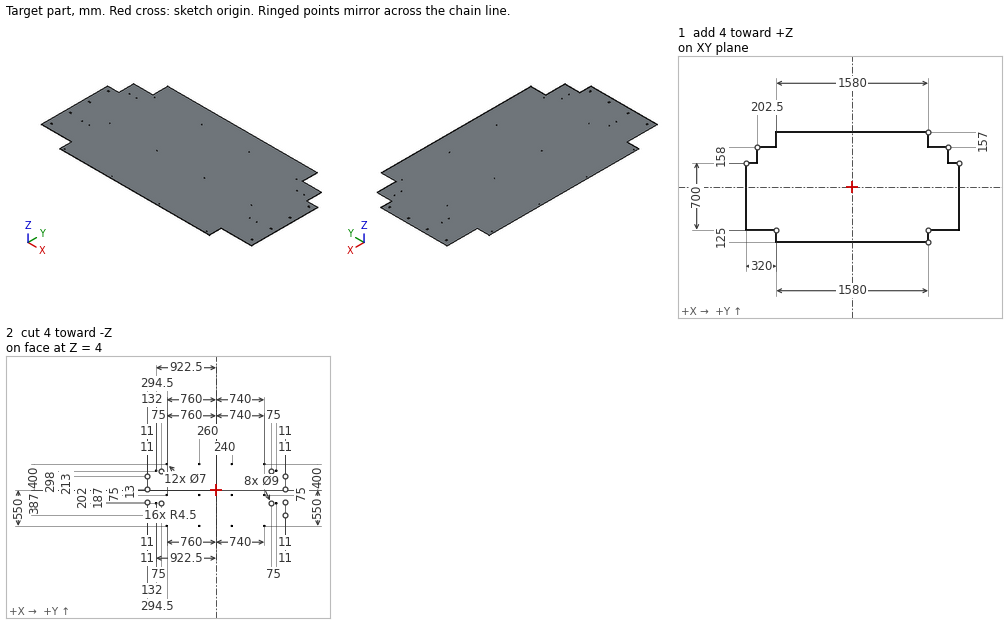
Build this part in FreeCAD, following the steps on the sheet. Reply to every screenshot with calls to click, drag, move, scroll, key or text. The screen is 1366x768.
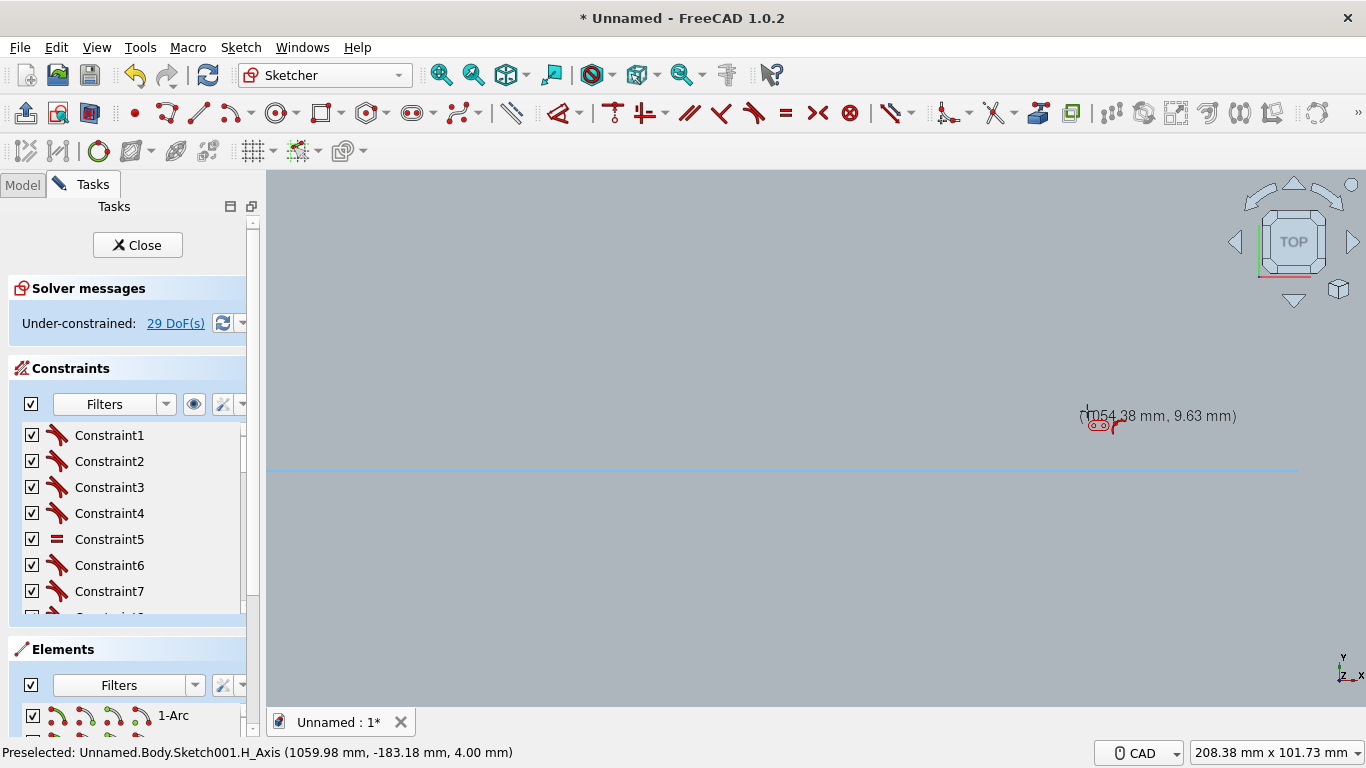
scroll(1087, 411, down, 14)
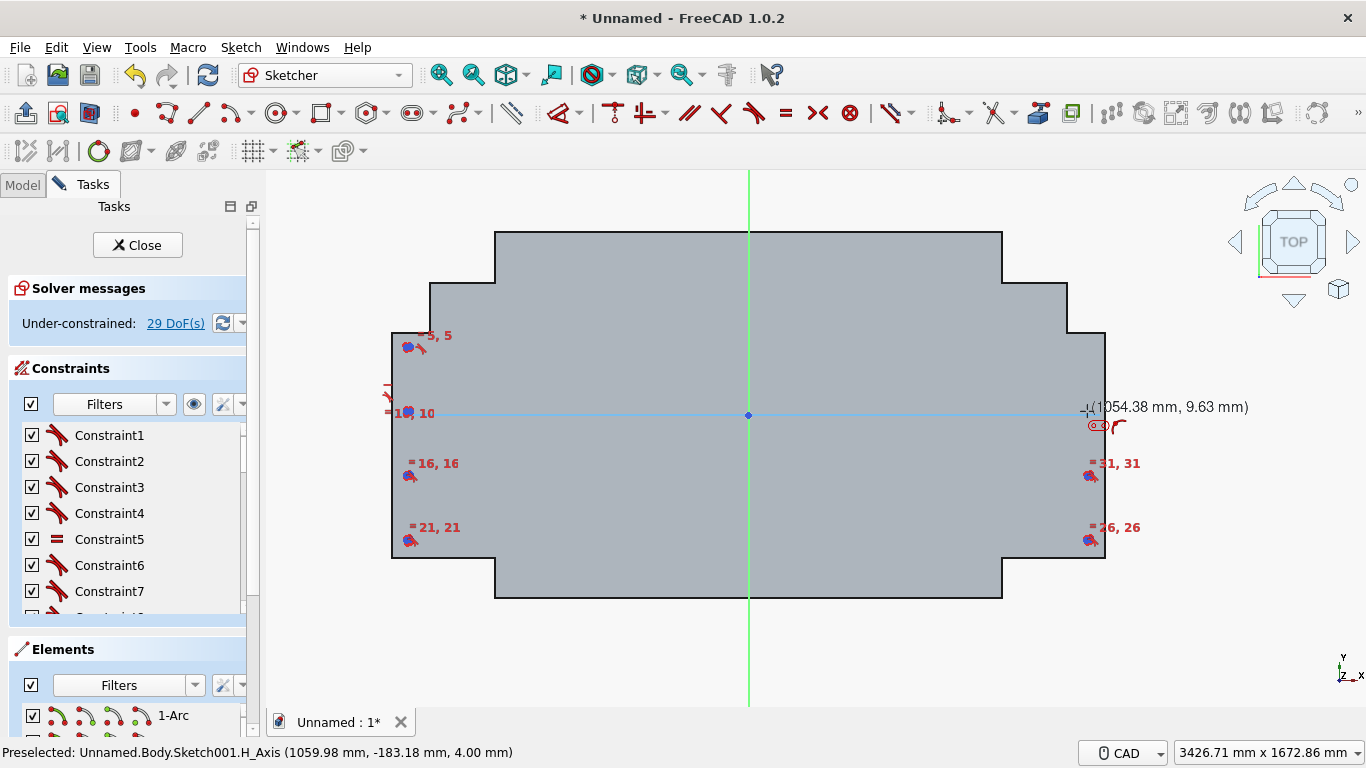
scroll(1087, 411, up, 7)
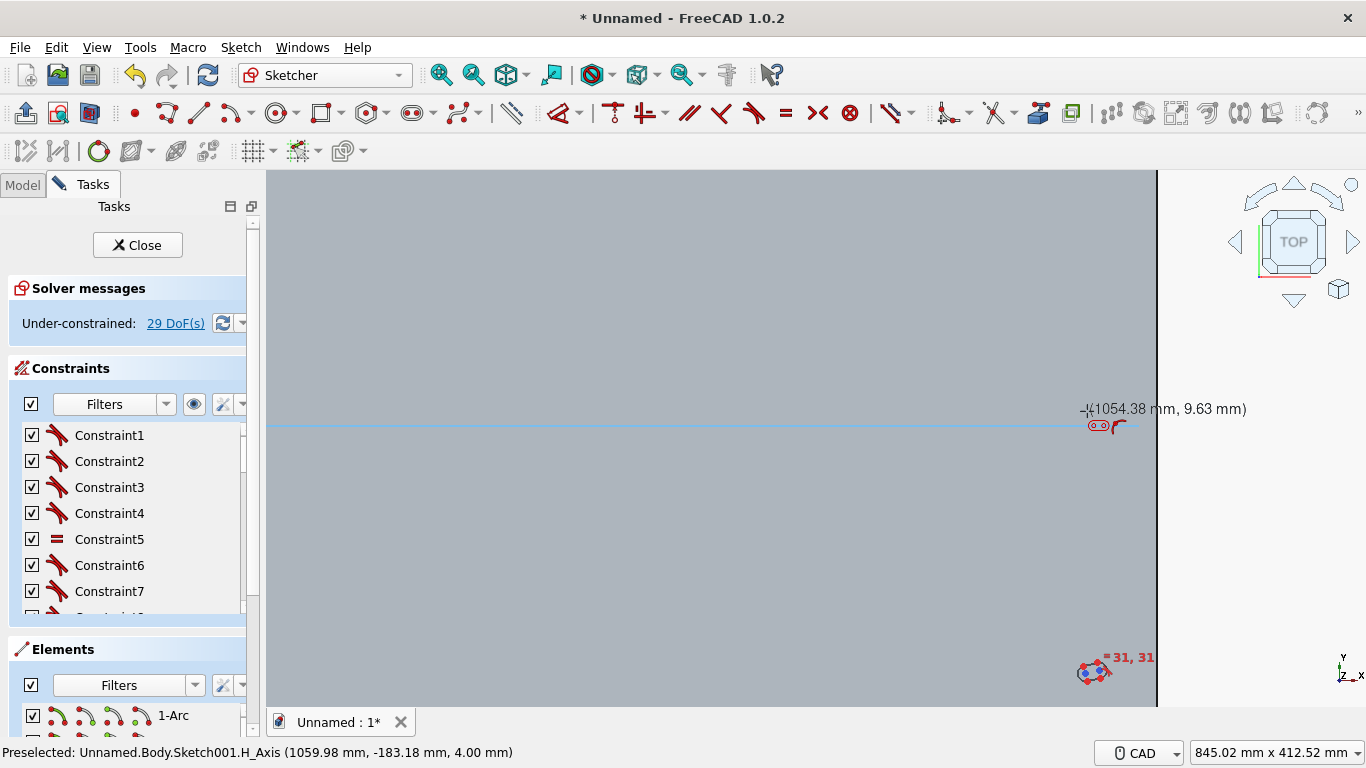
click(1085, 409)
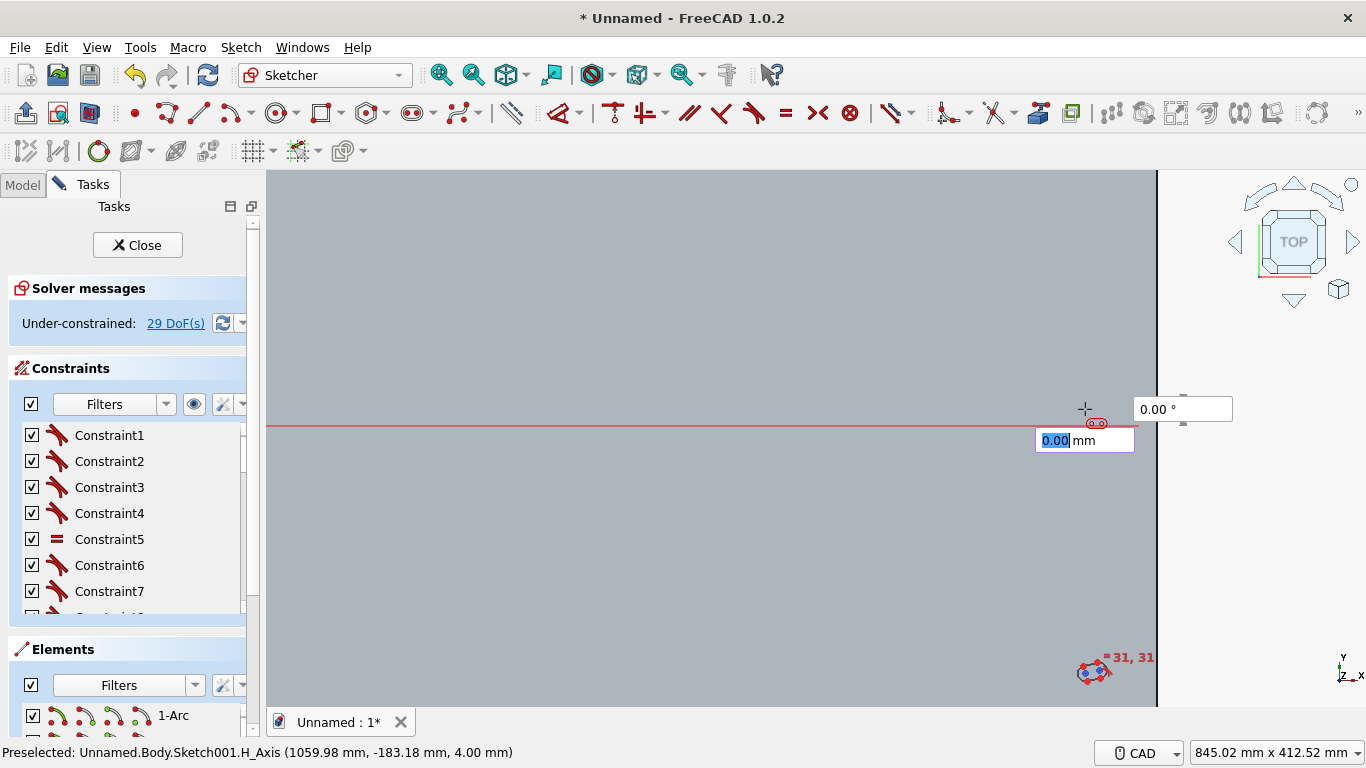
click(1099, 409)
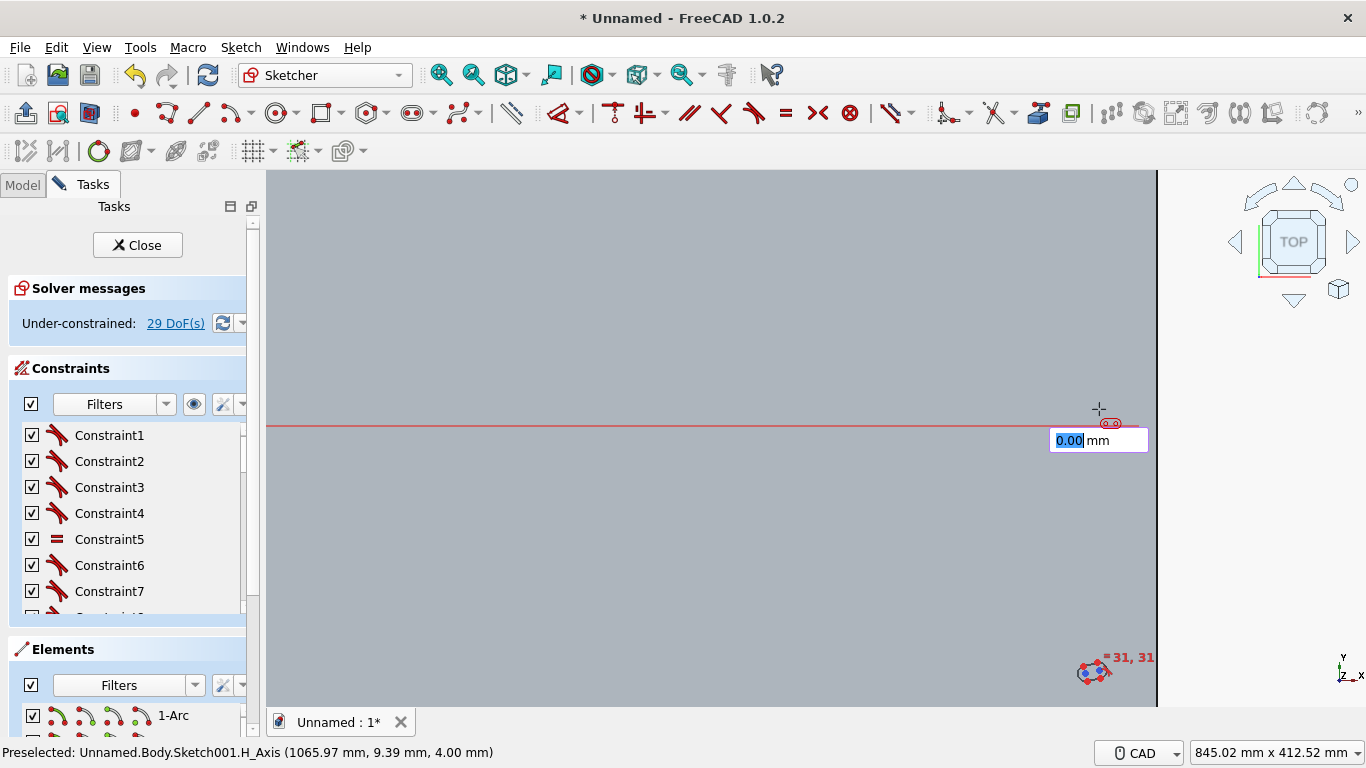
scroll(1092, 403, up, 5)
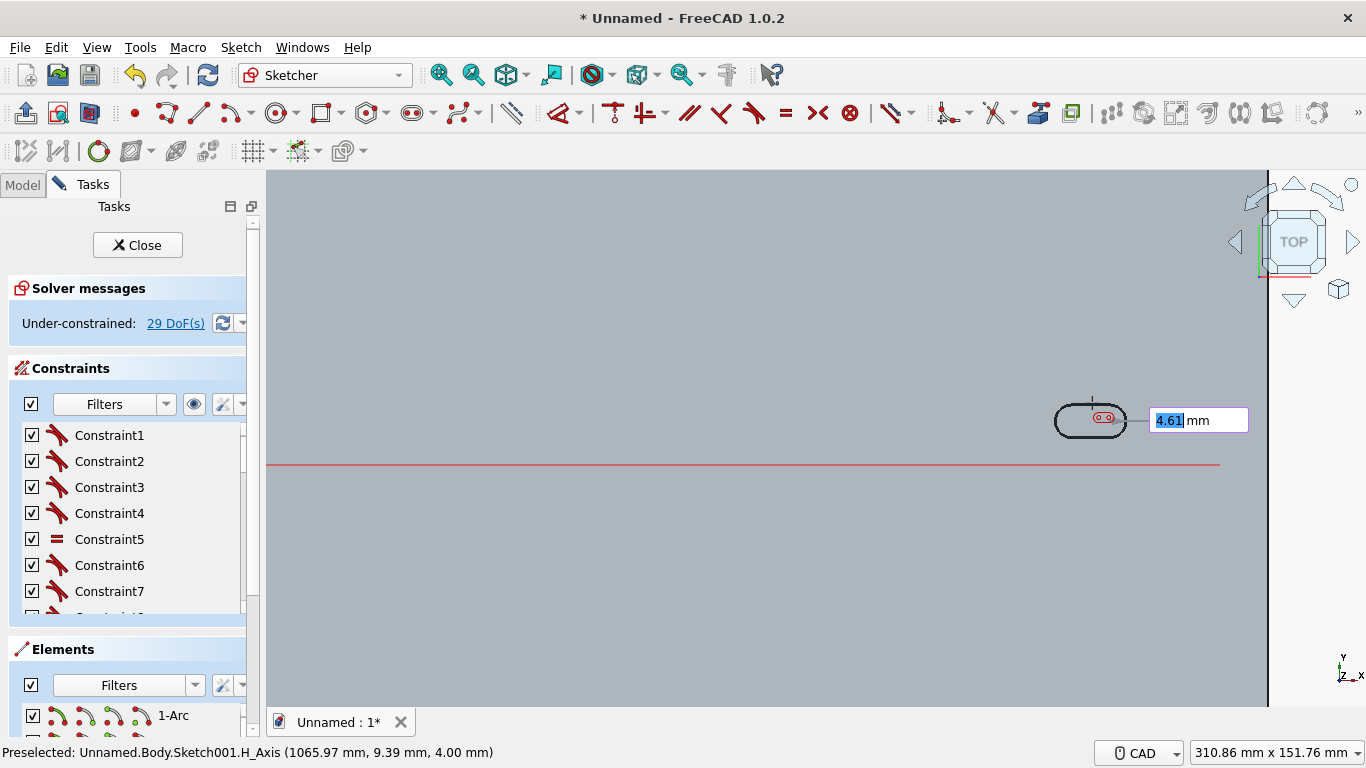
click(1091, 403)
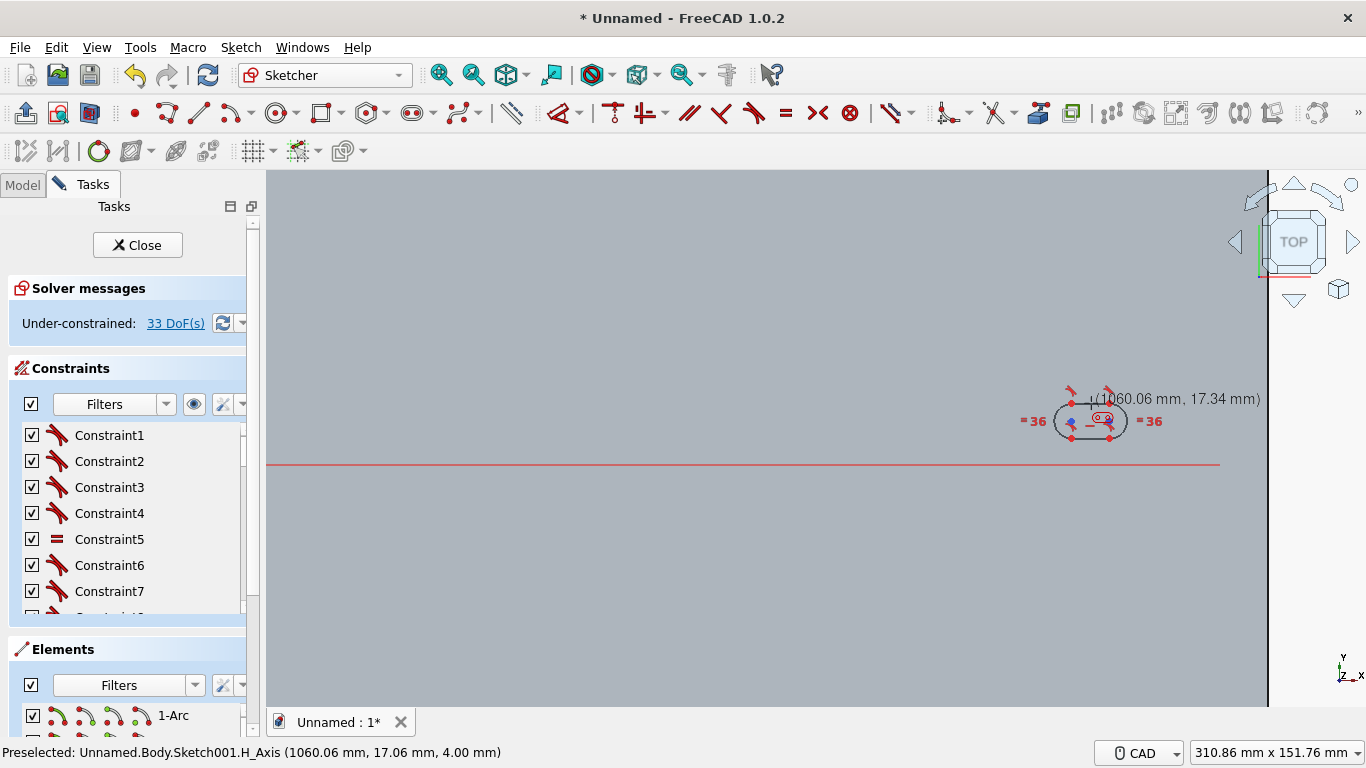
scroll(1087, 409, down, 12)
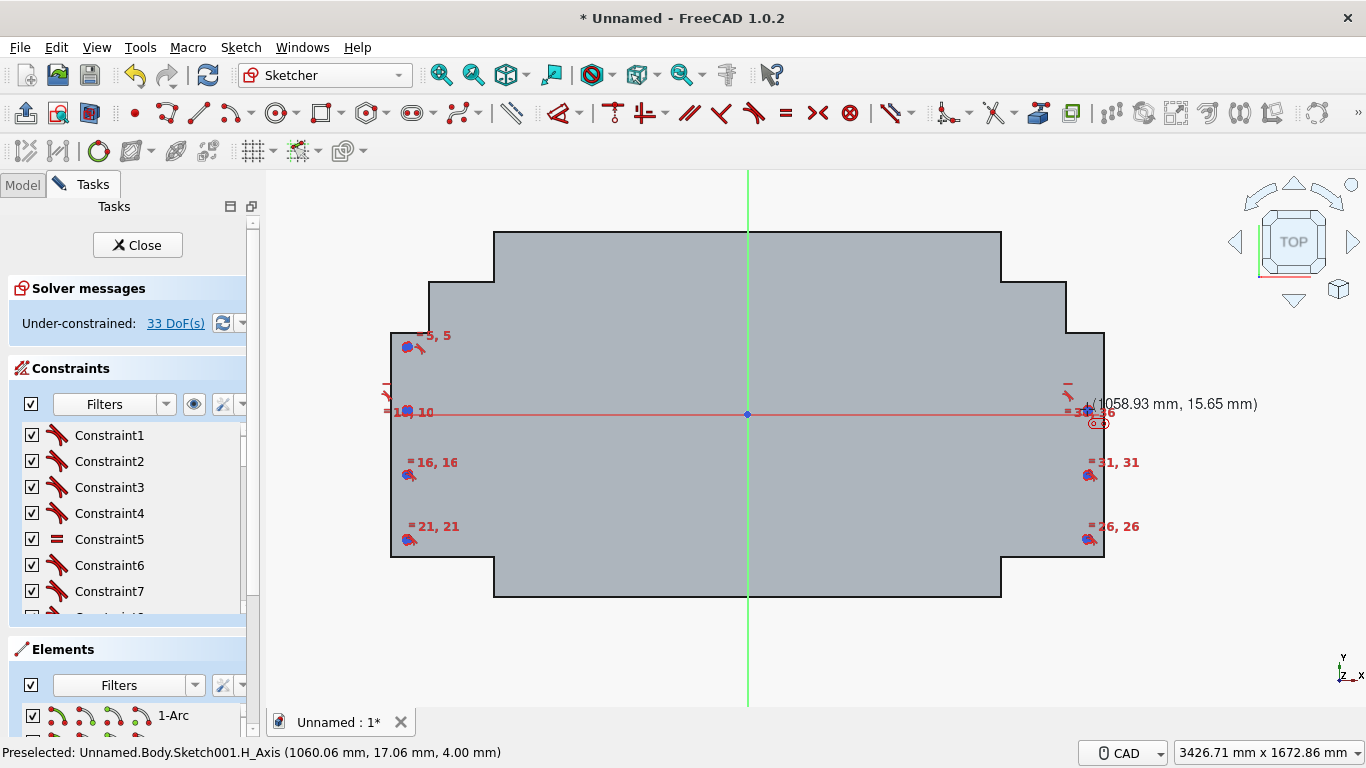
scroll(1086, 346, up, 14)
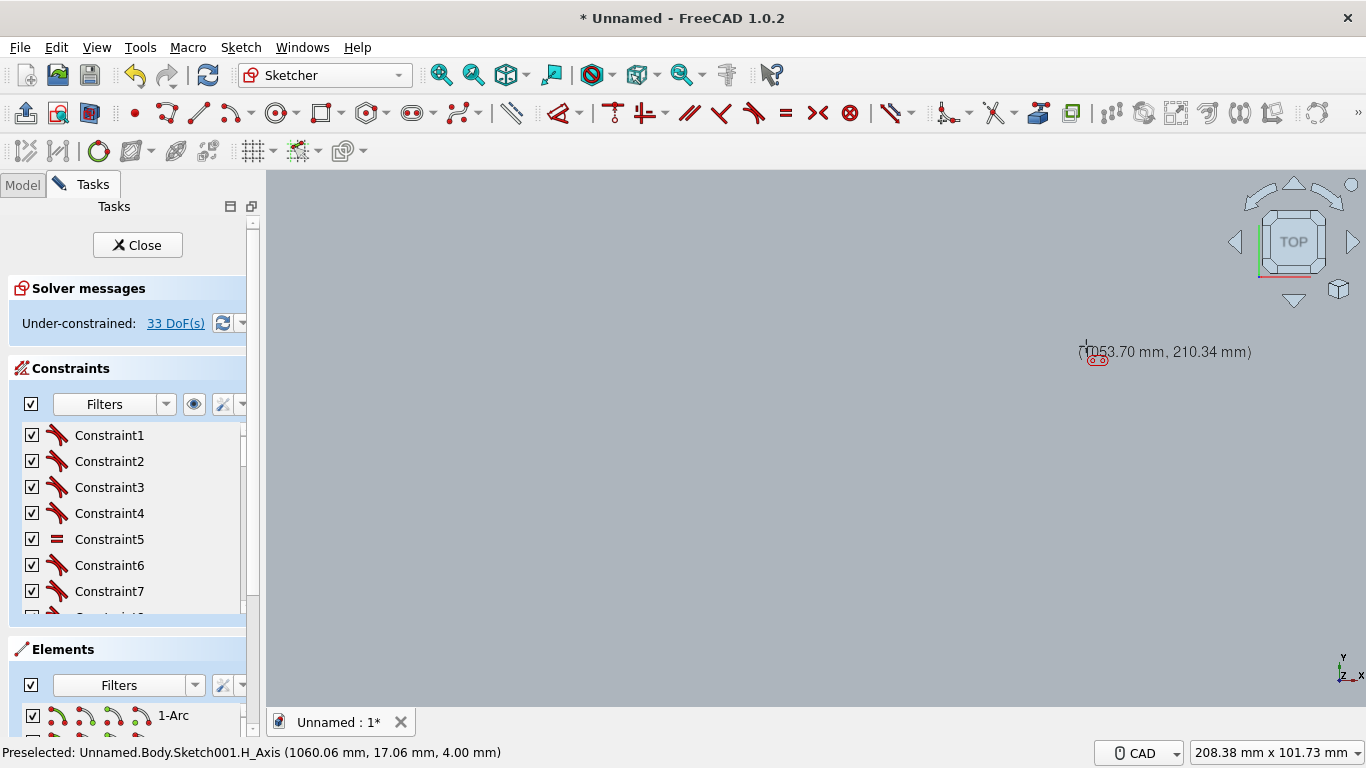
scroll(1086, 346, down, 14)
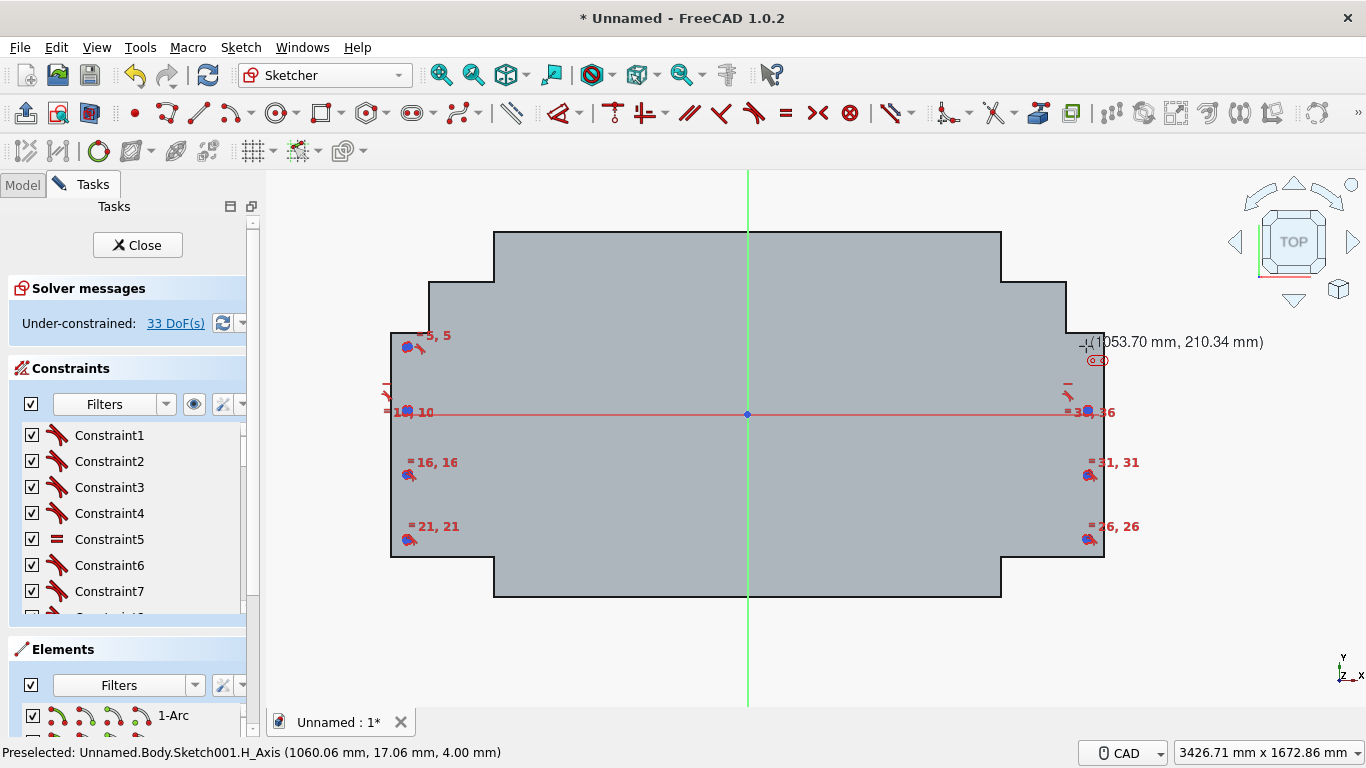
click(1086, 346)